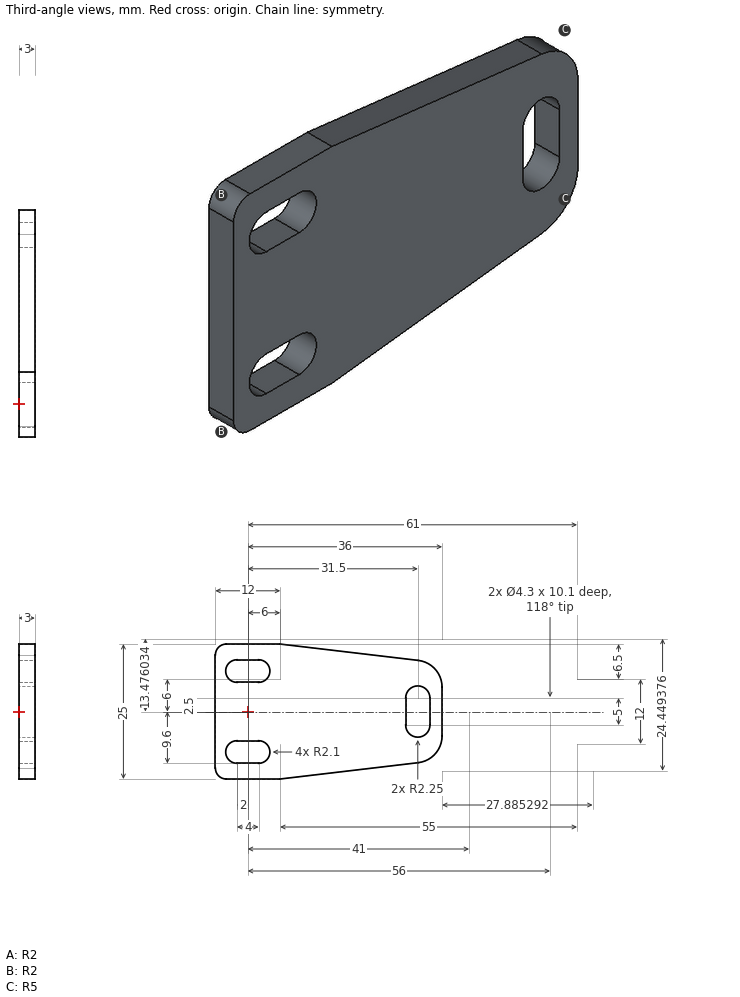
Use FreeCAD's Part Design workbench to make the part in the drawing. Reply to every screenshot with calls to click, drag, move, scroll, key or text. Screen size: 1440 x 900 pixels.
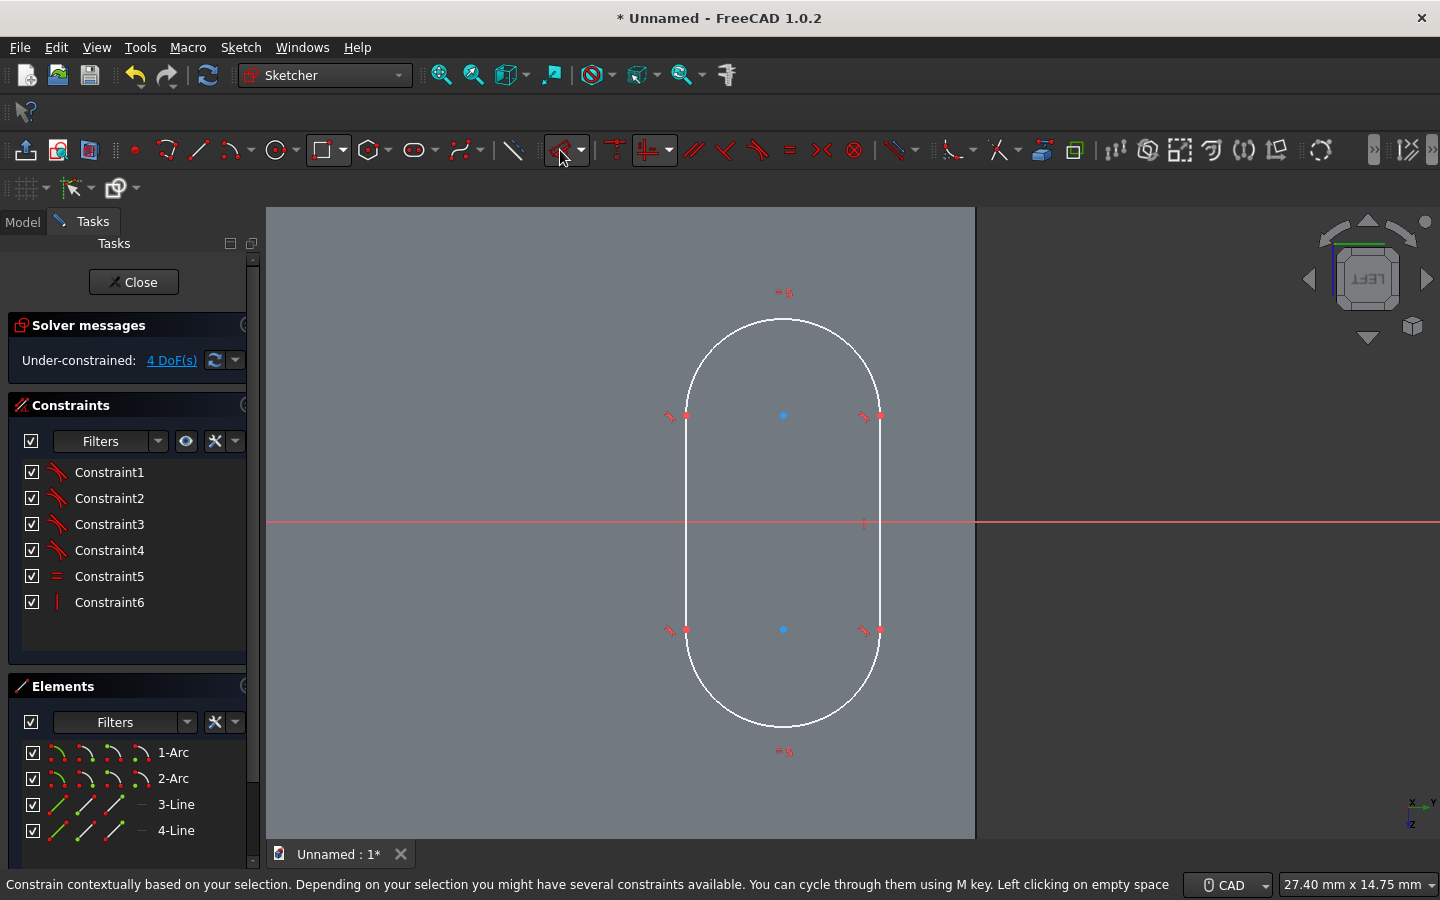
click(726, 708)
click(707, 734)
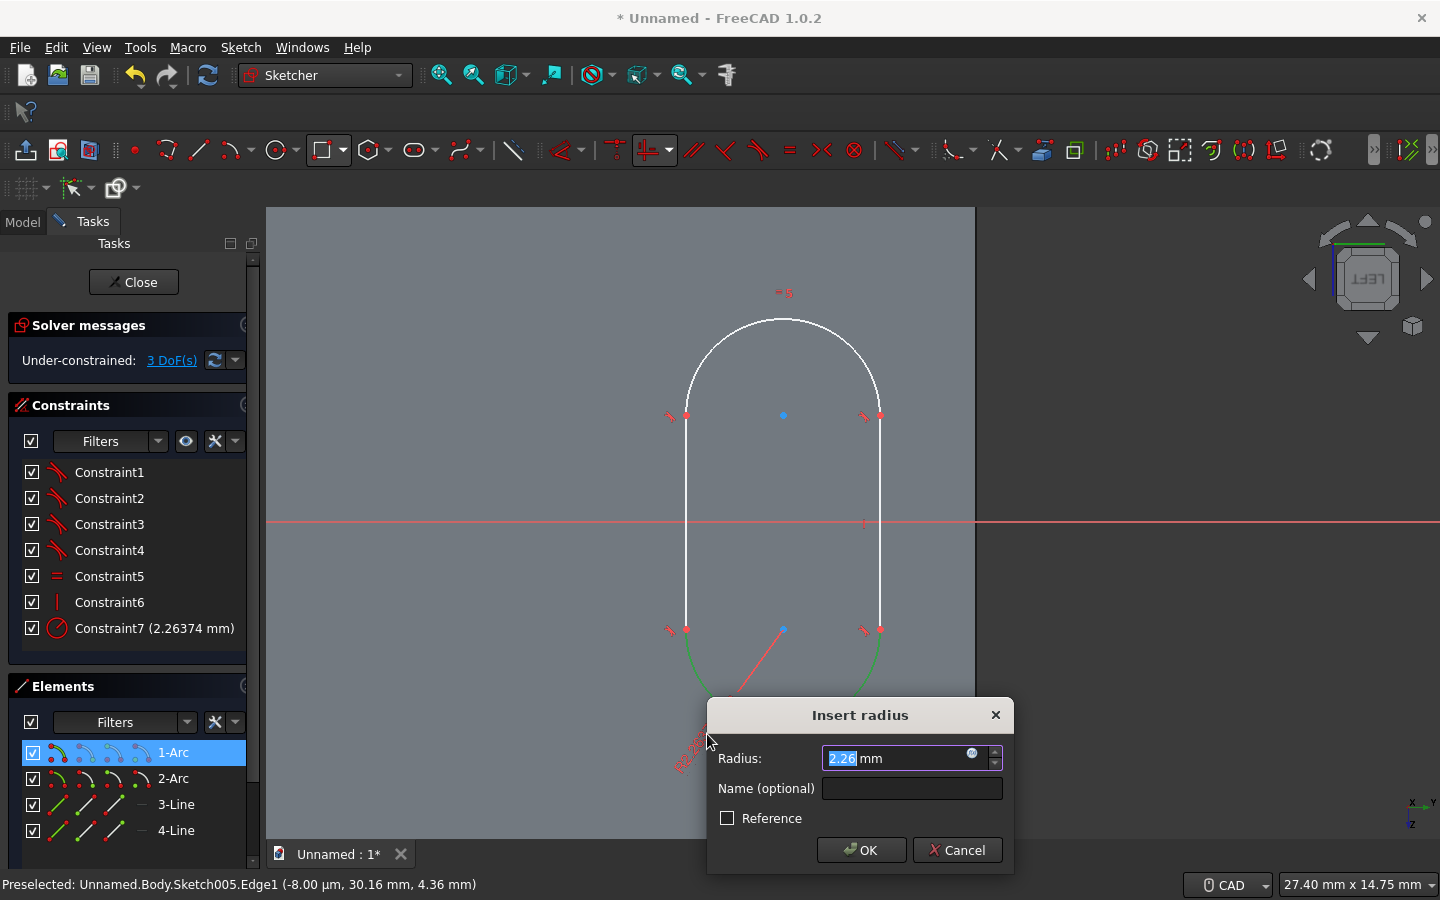
text(2.25)
key(Return)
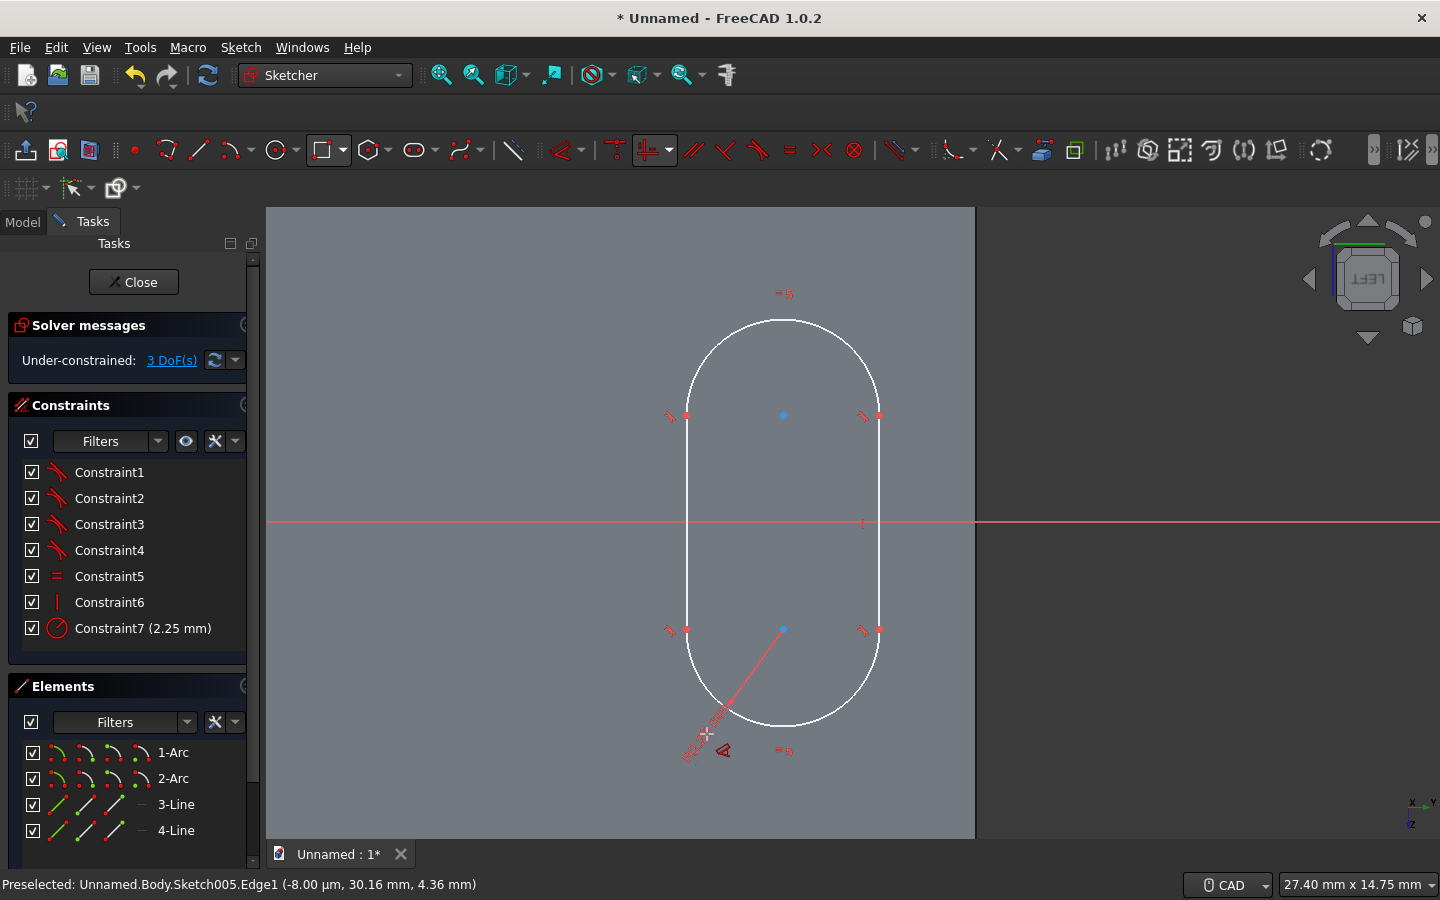
click(687, 566)
click(653, 474)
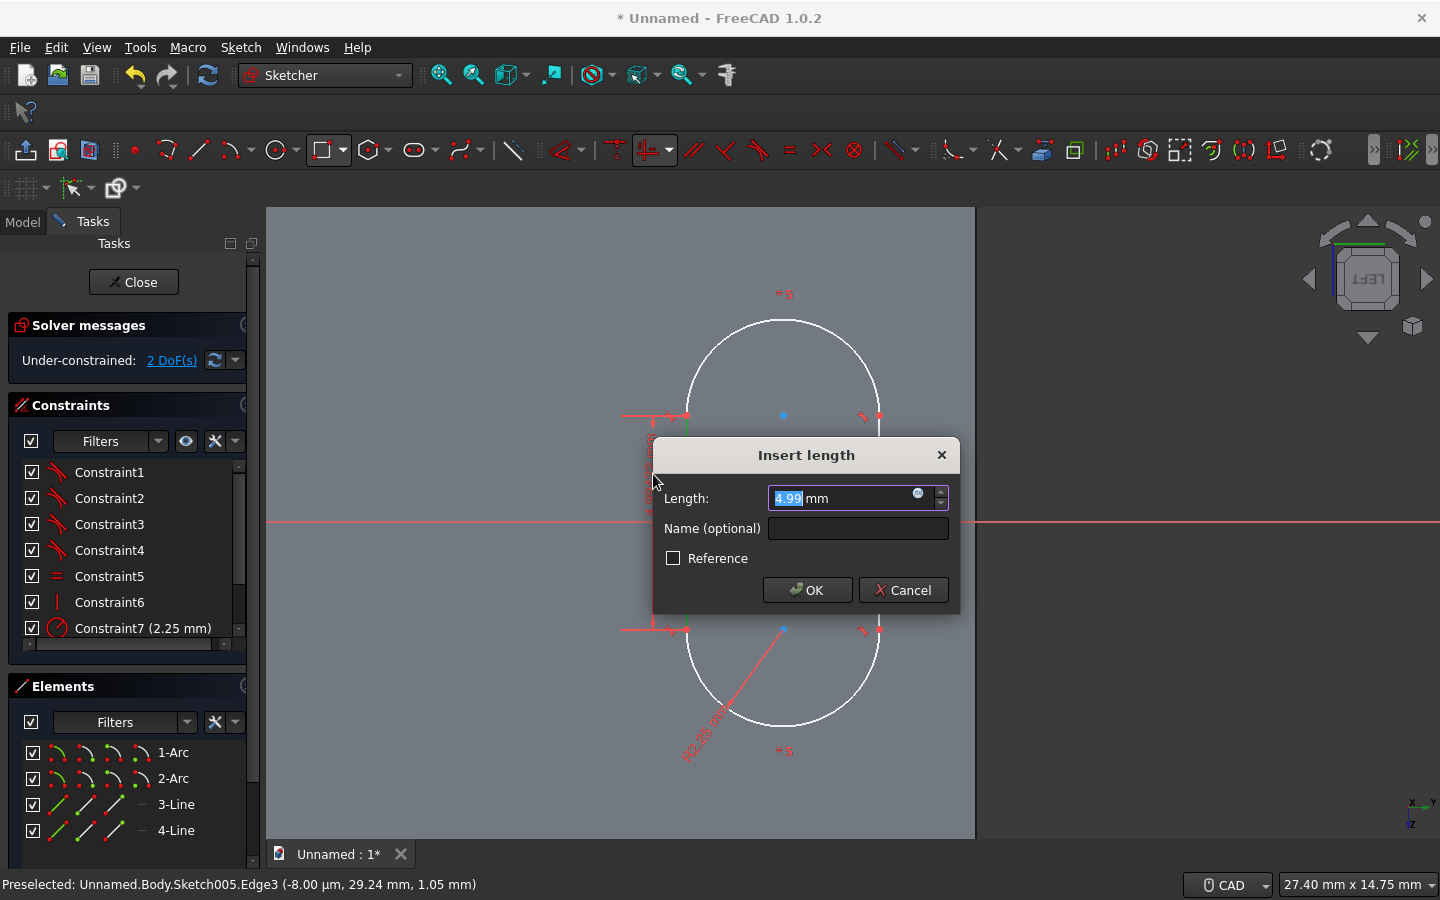
text(5)
key(Return)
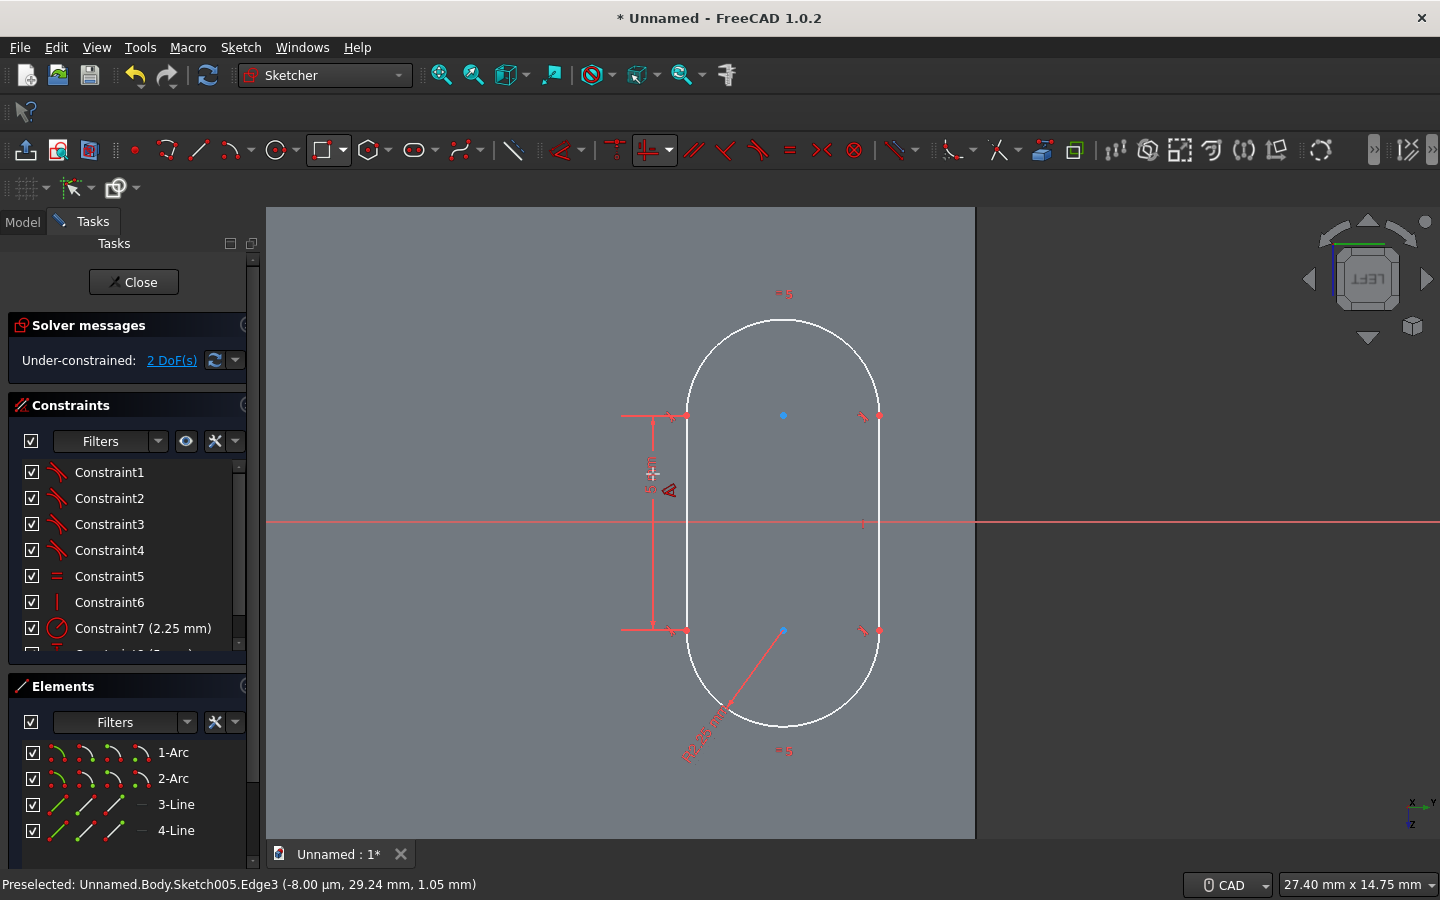
click(687, 630)
click(721, 576)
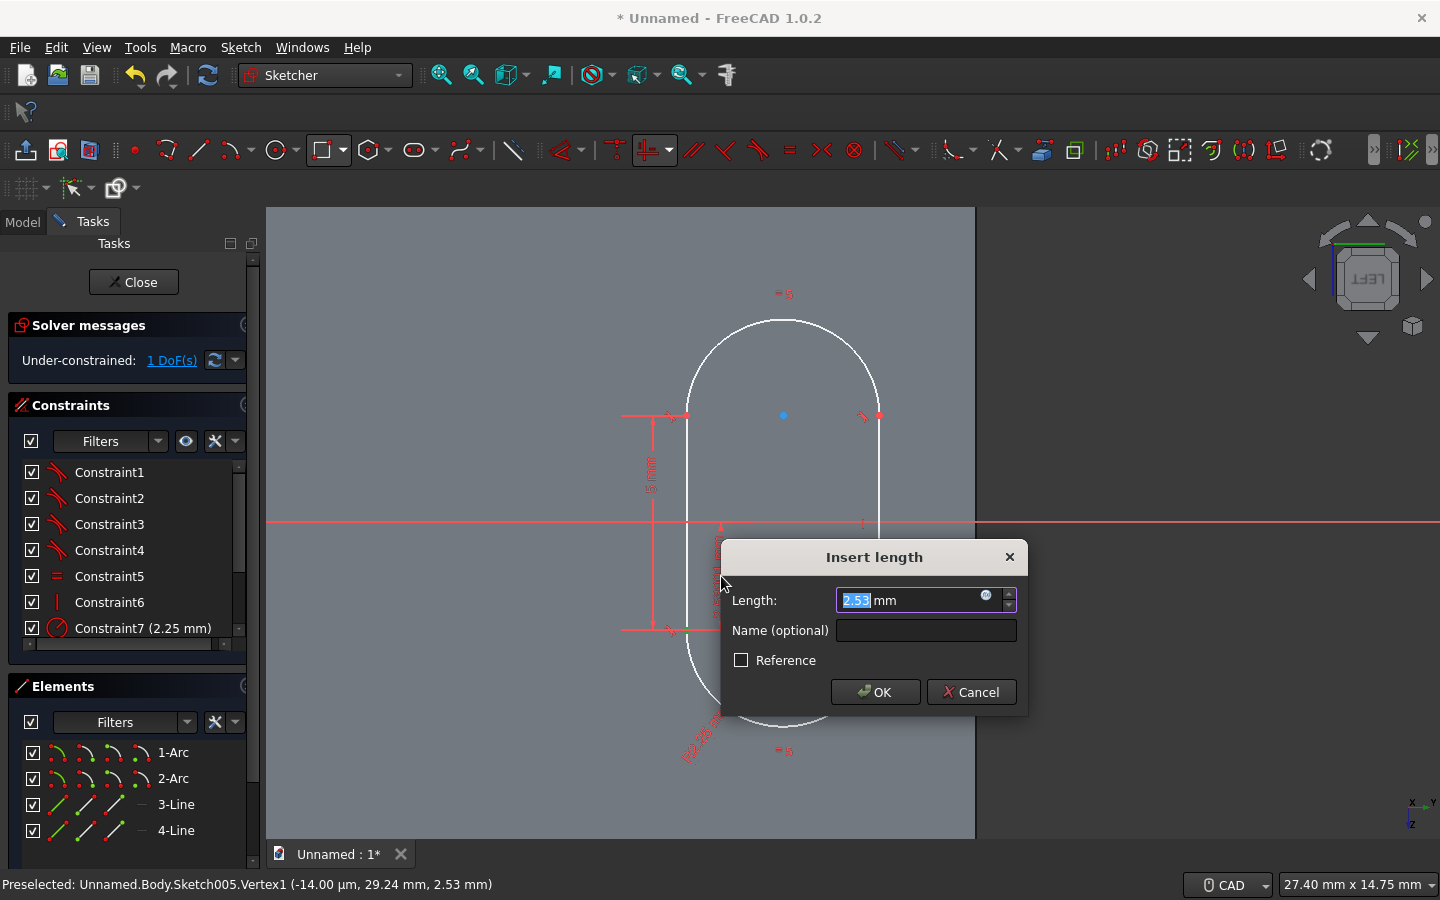
text(2.5)
key(Return)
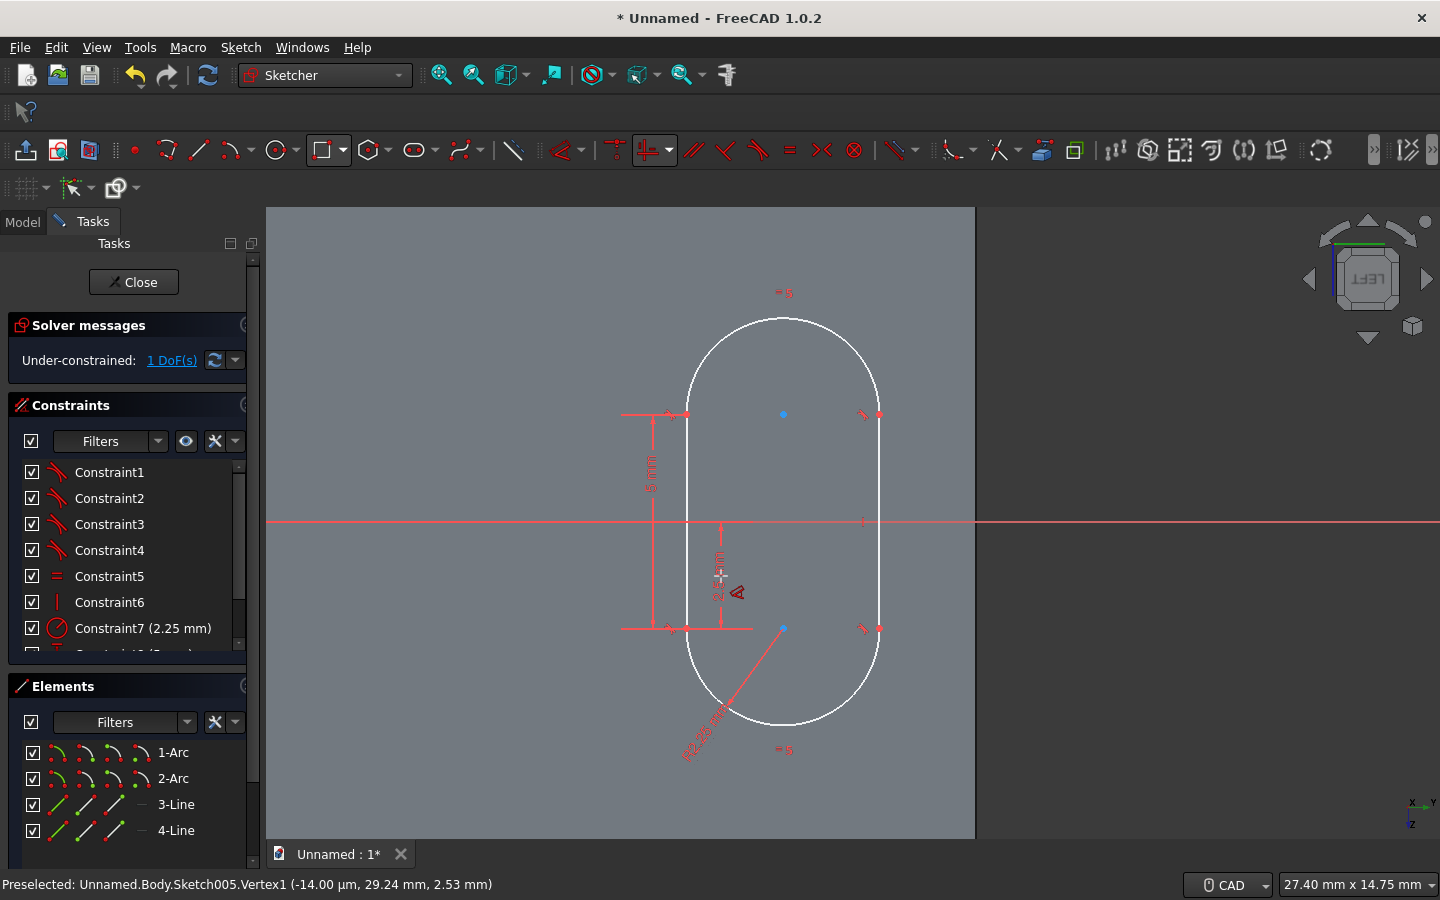
click(783, 629)
click(538, 663)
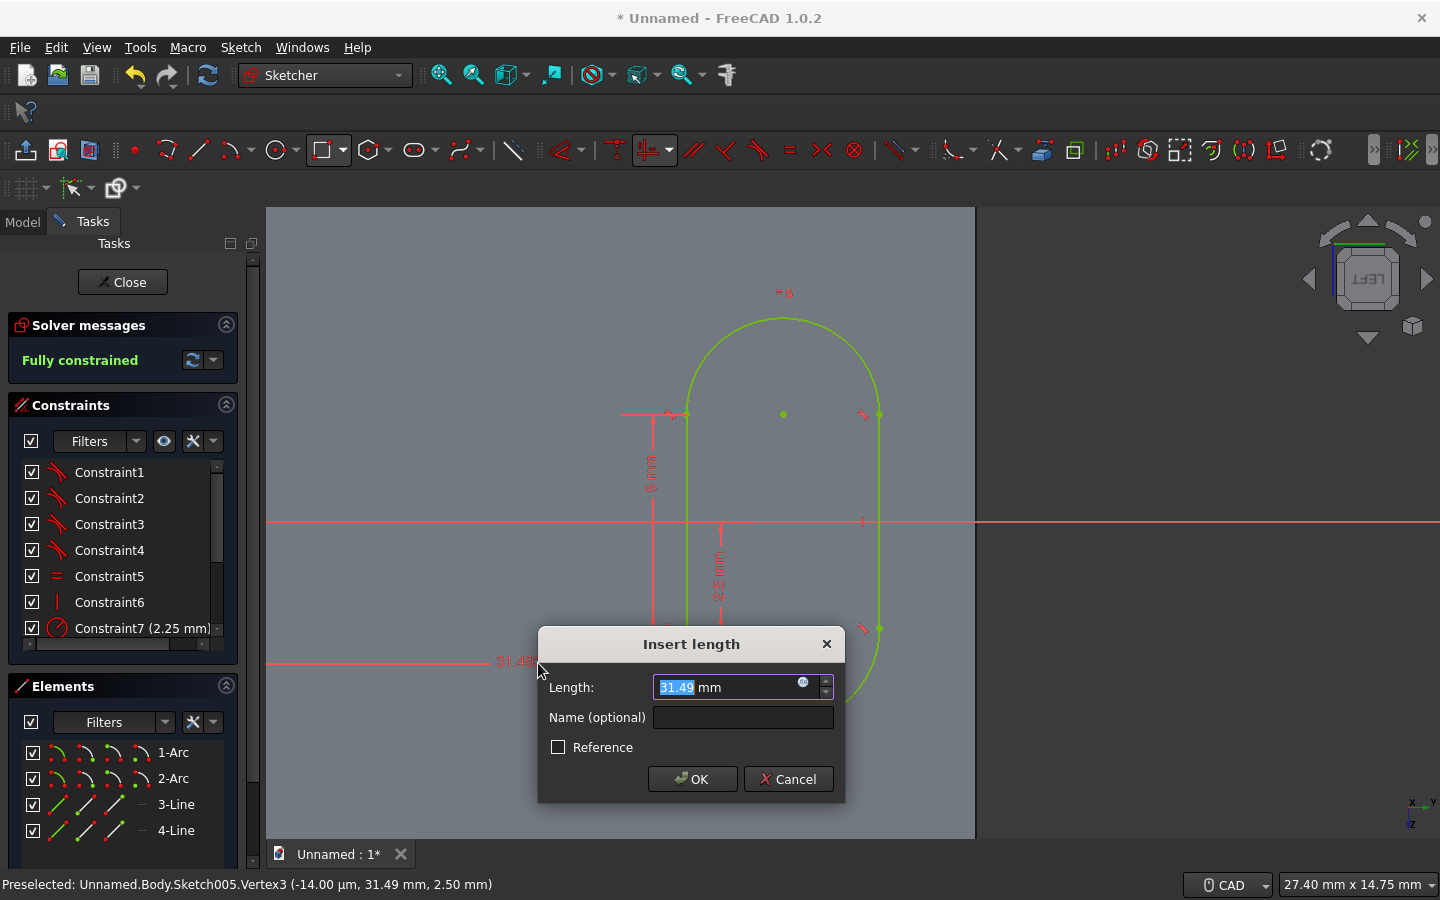
text(31.5)
key(Return)
key(Escape)